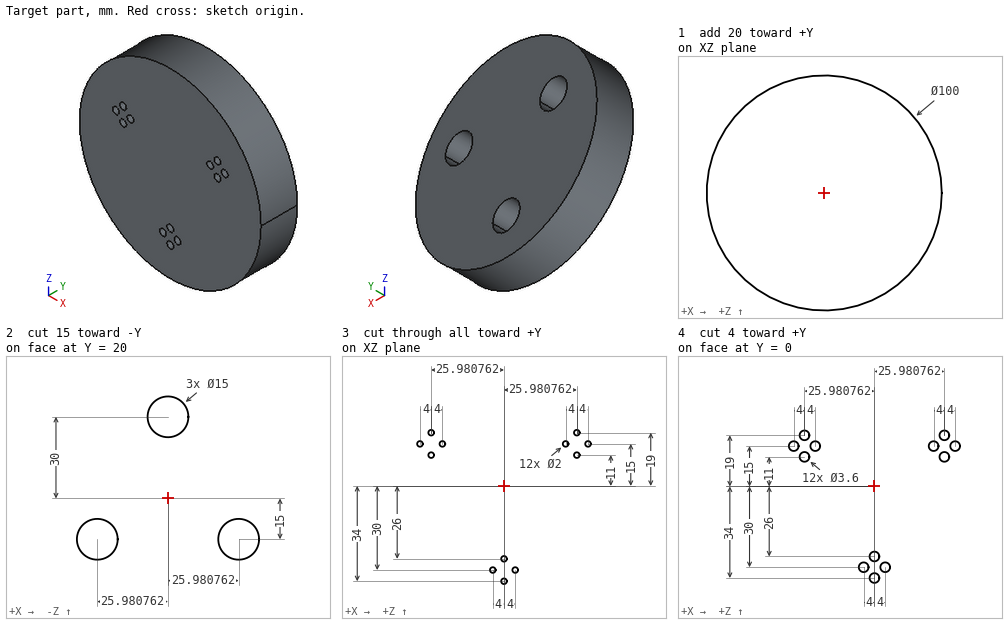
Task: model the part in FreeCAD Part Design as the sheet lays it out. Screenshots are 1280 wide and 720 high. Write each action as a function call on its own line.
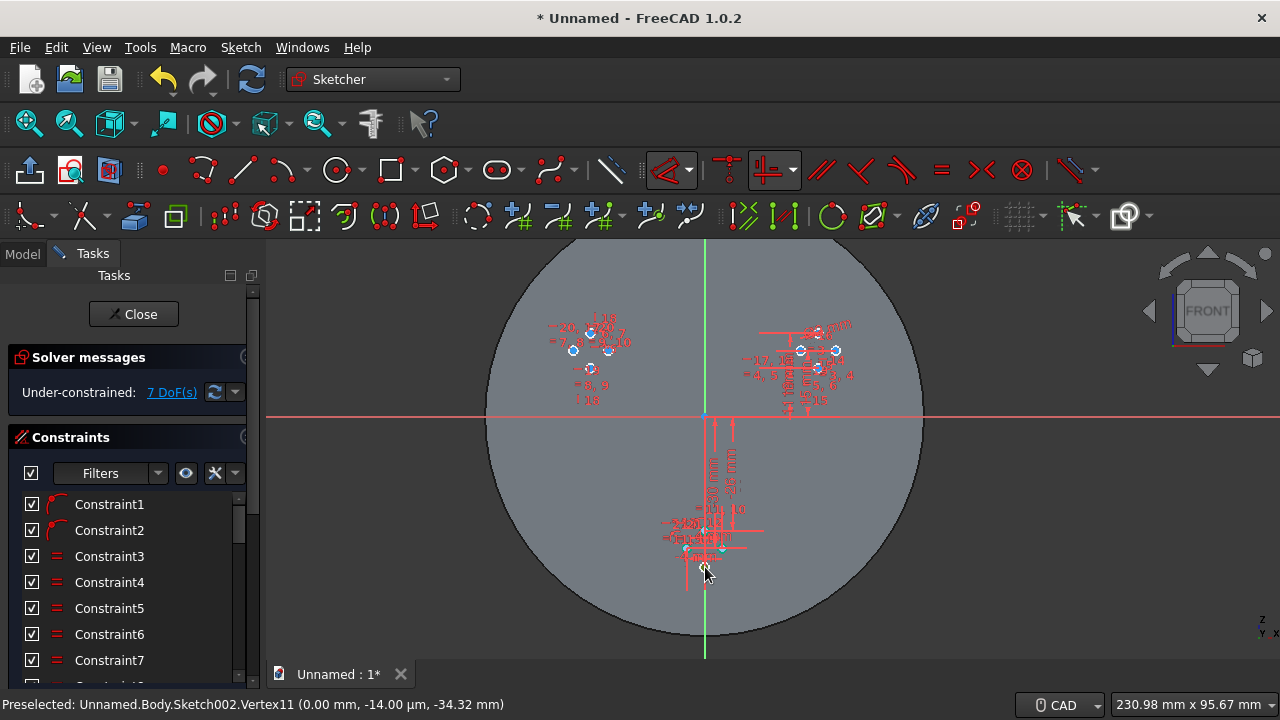
key(i)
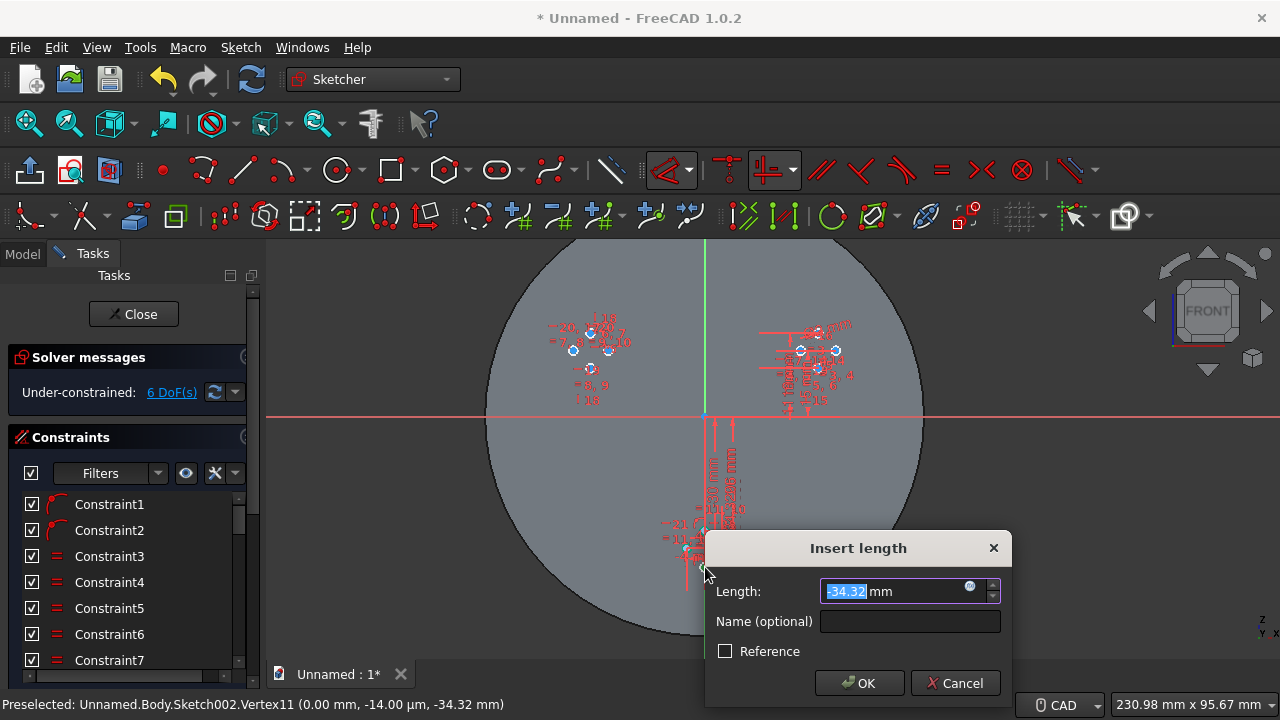
text(-34)
key(Return)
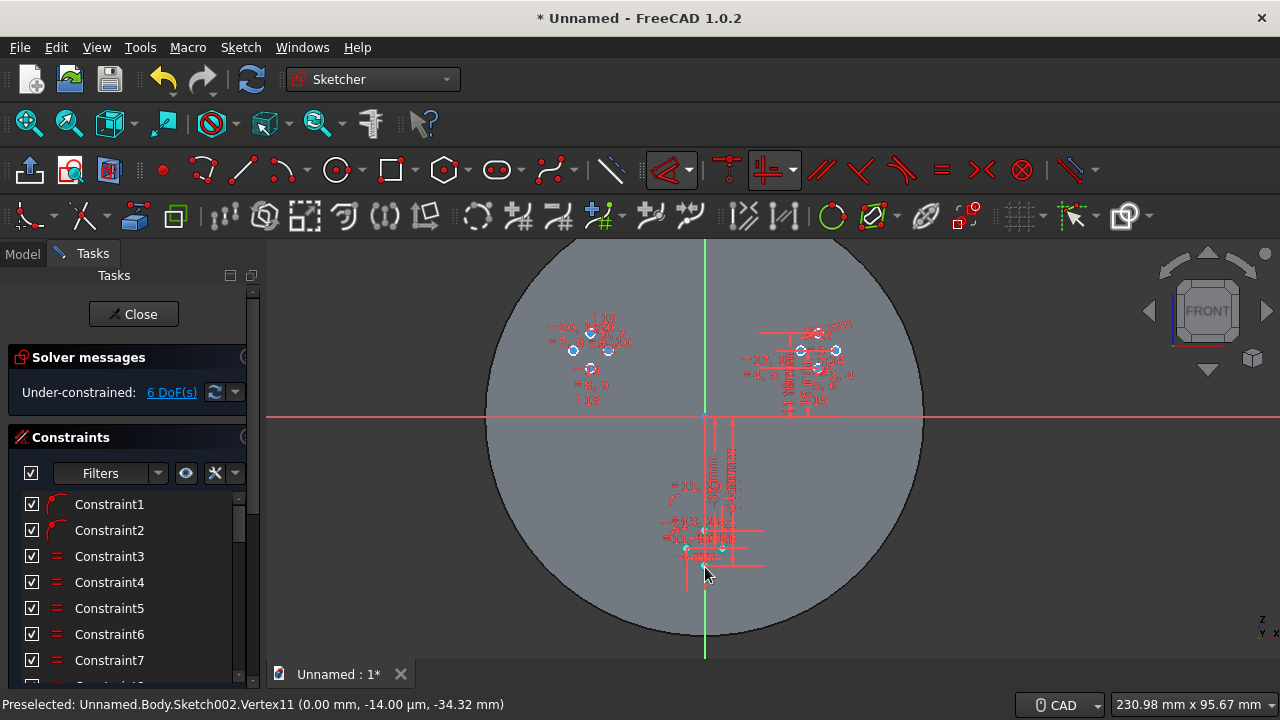
scroll(818, 333, up, 5)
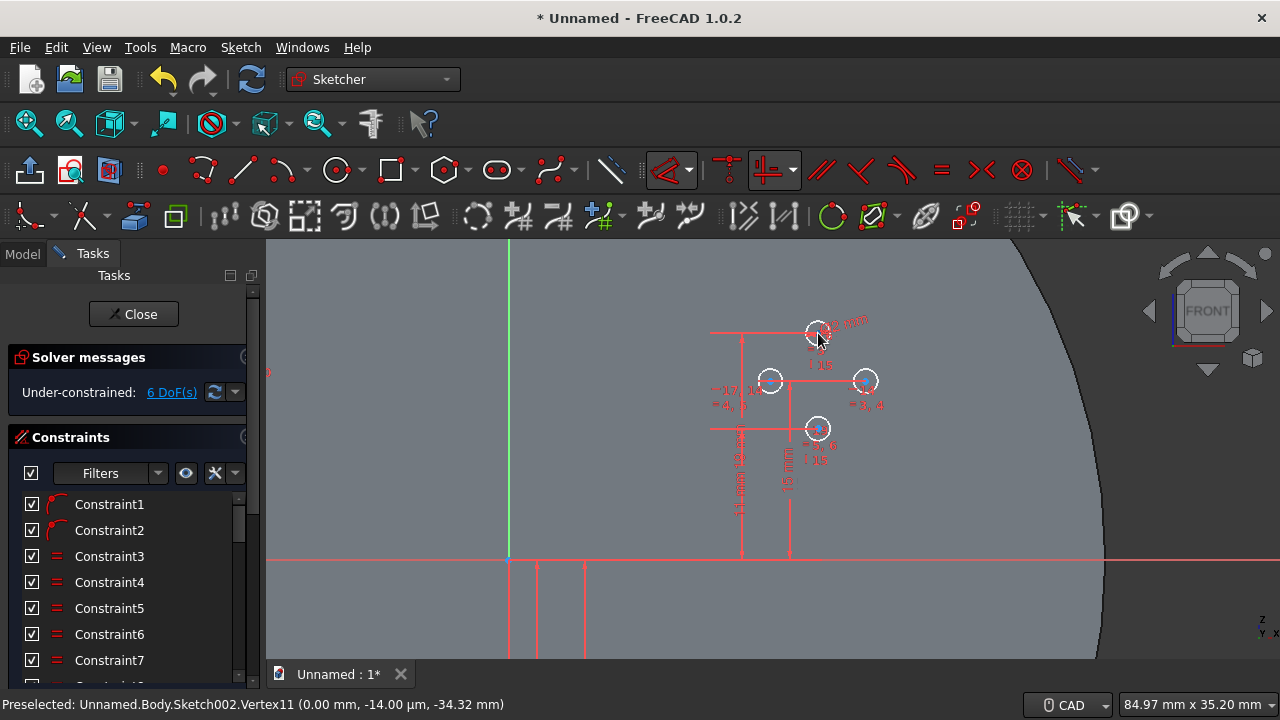
click(818, 333)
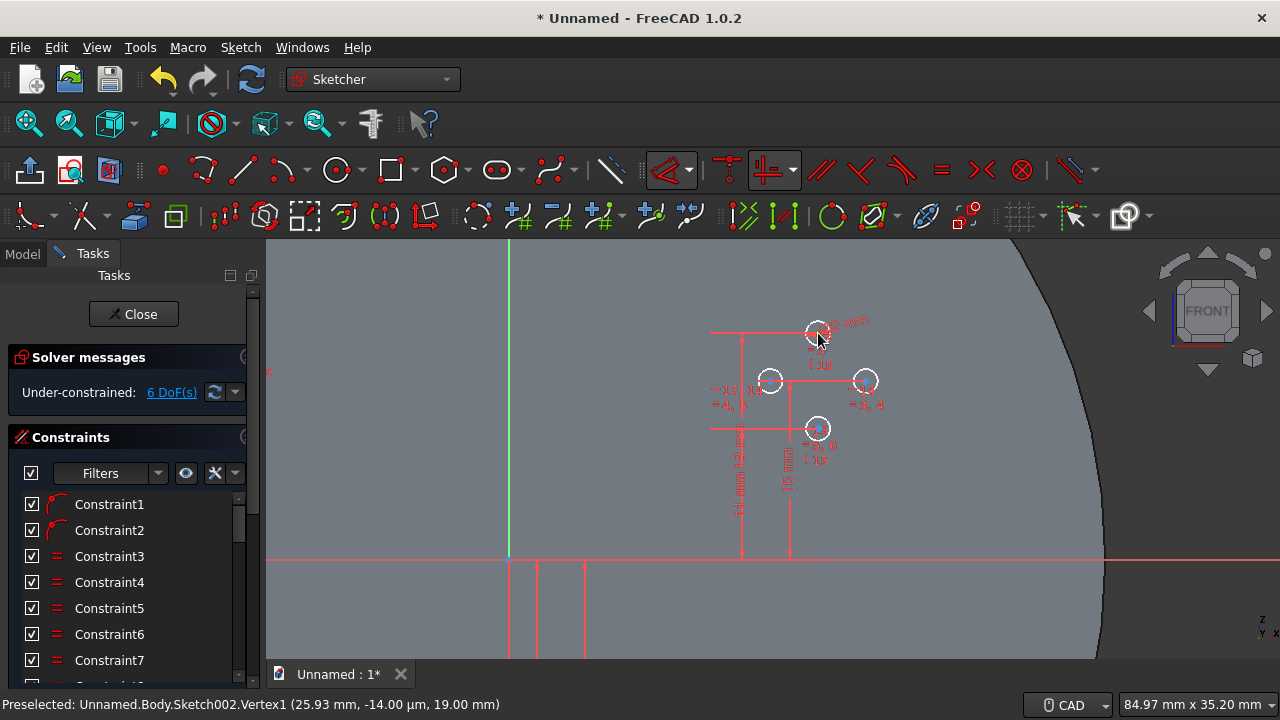
click(866, 381)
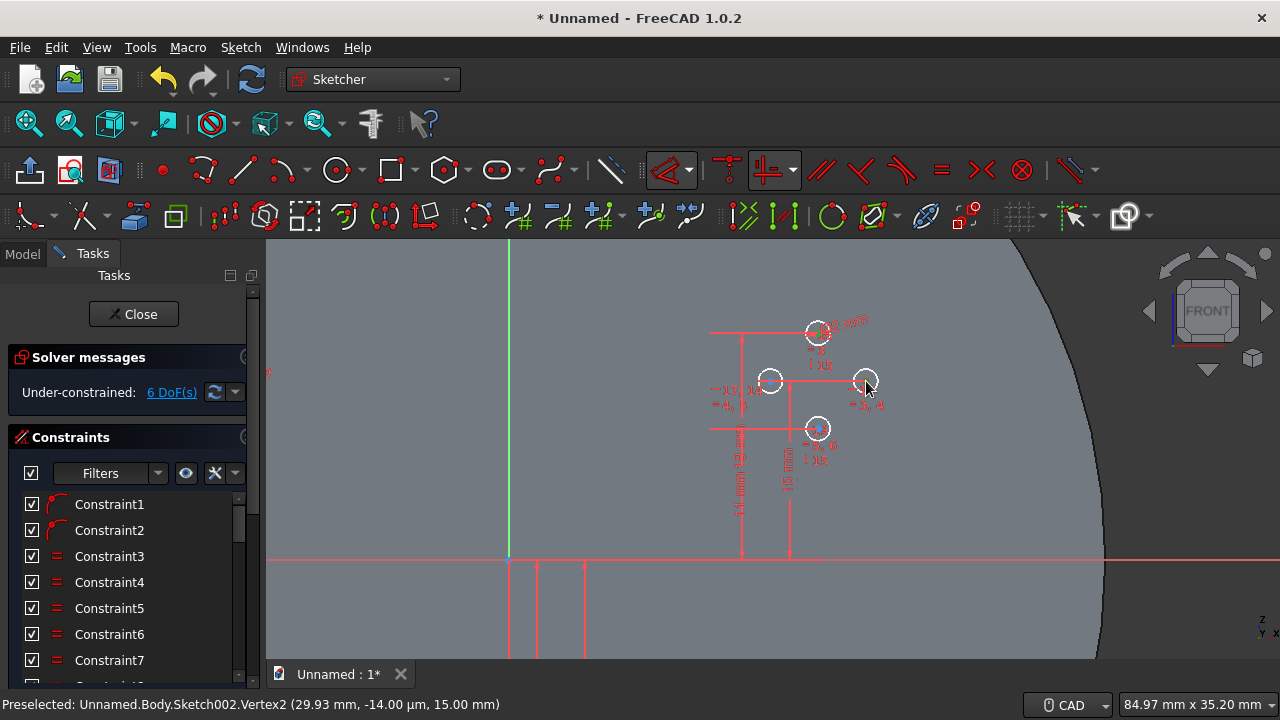
click(692, 170)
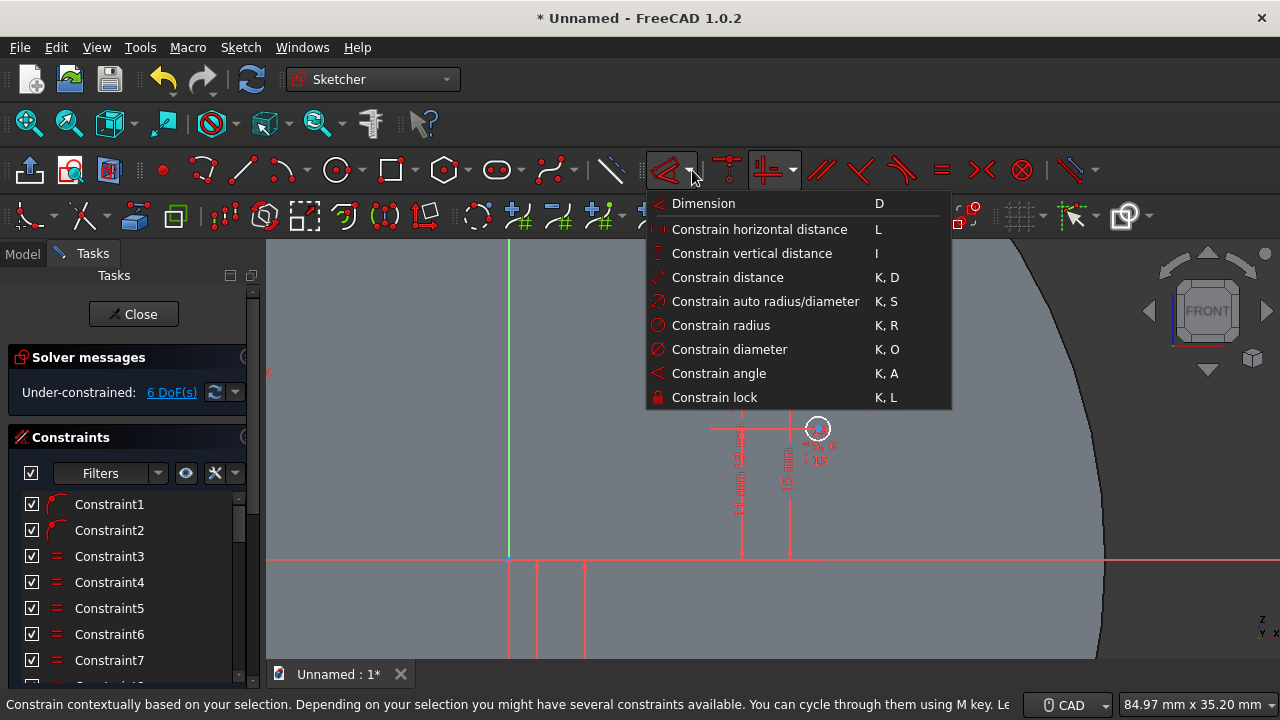
click(799, 229)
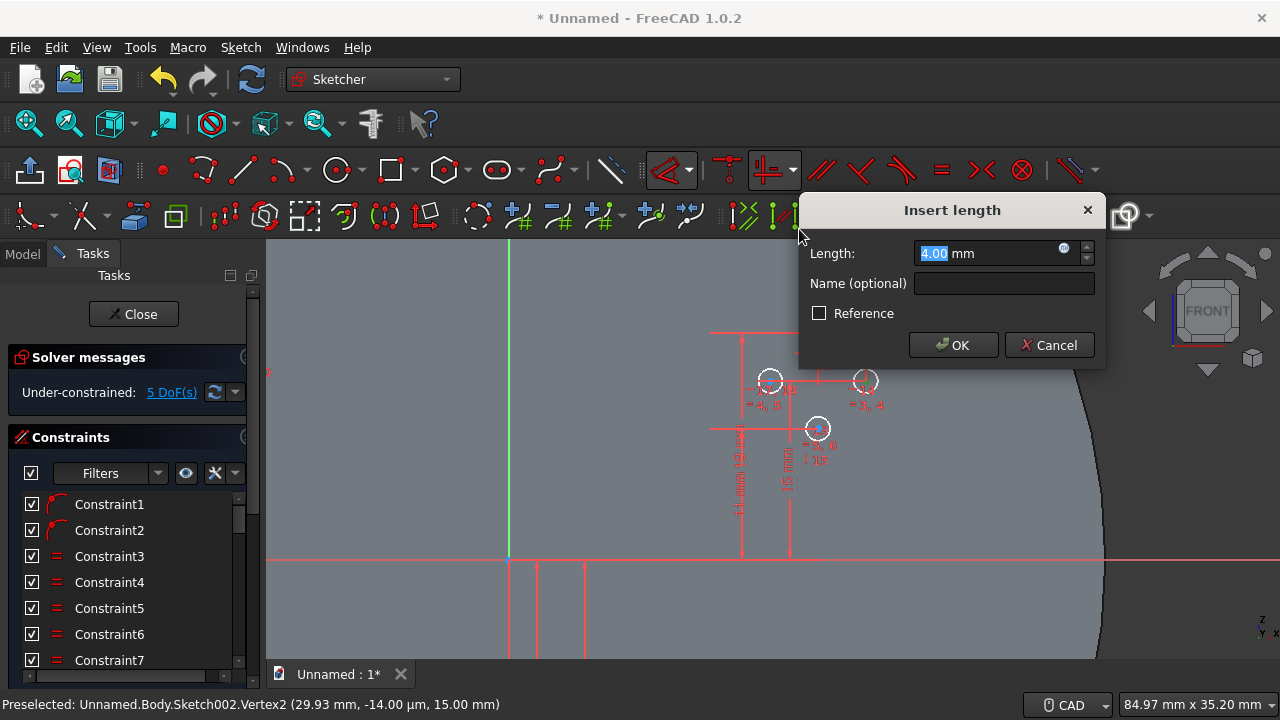
text(4)
key(Return)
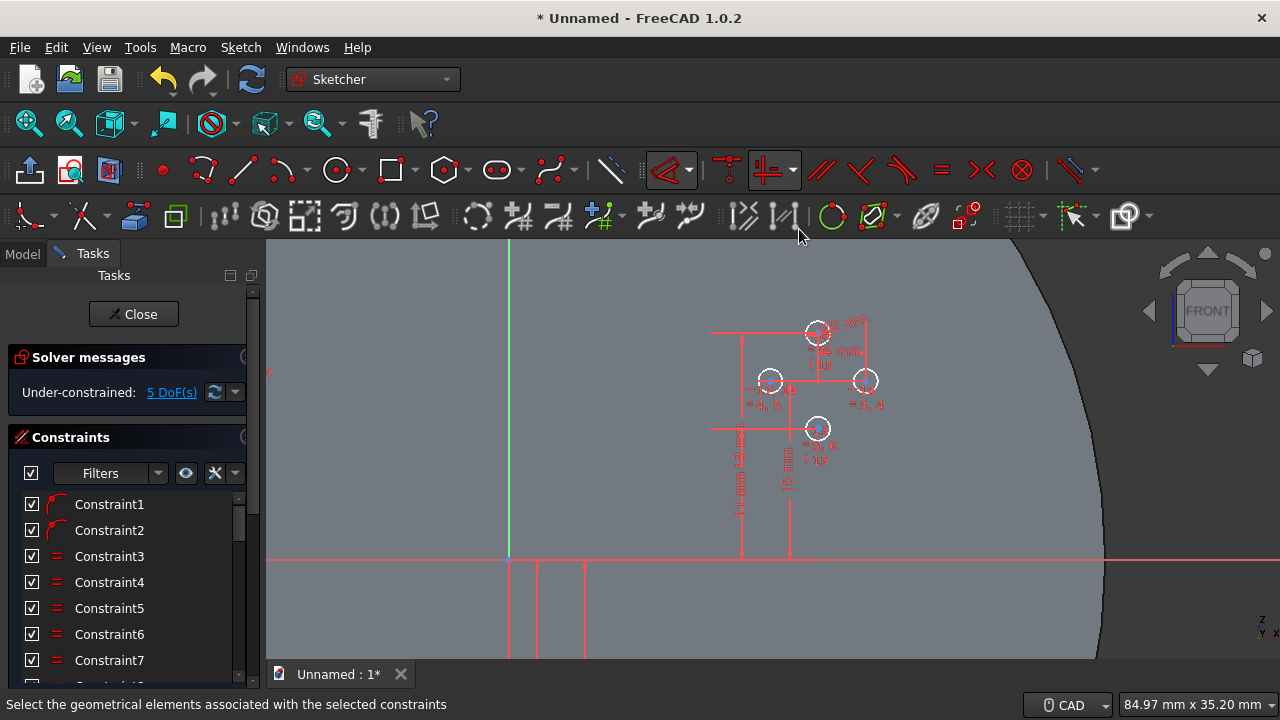
click(818, 333)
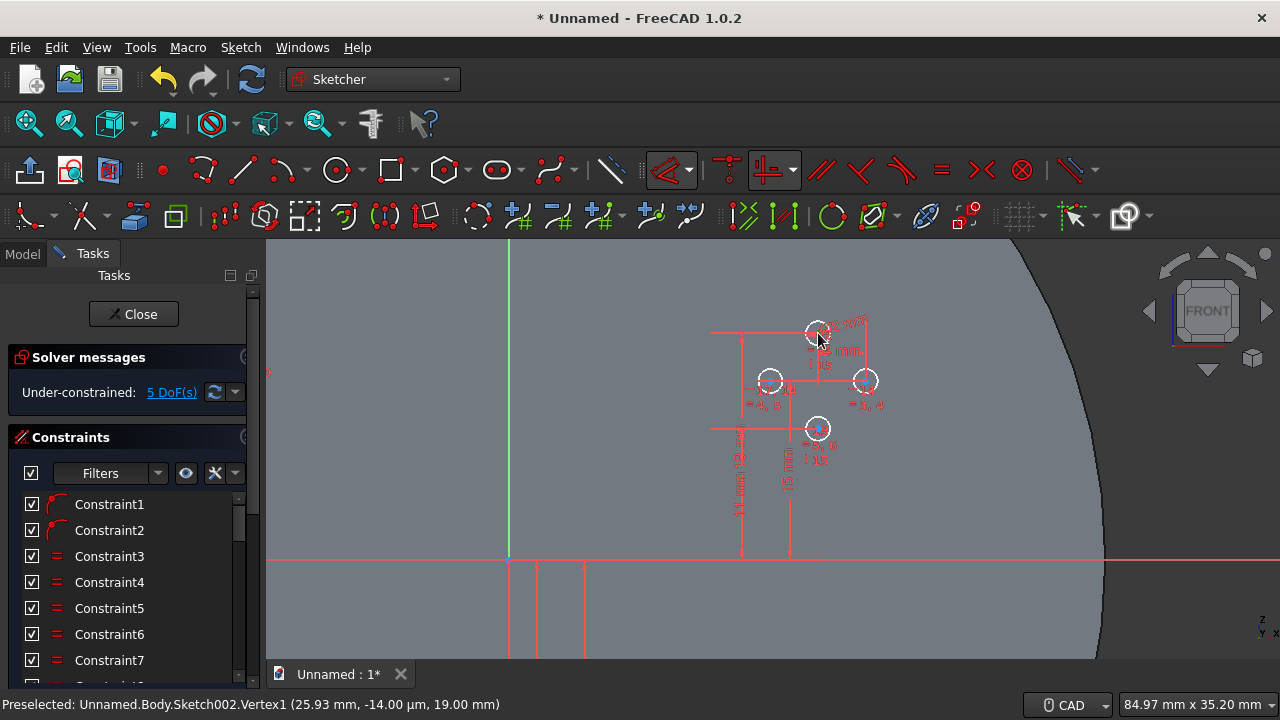
click(770, 381)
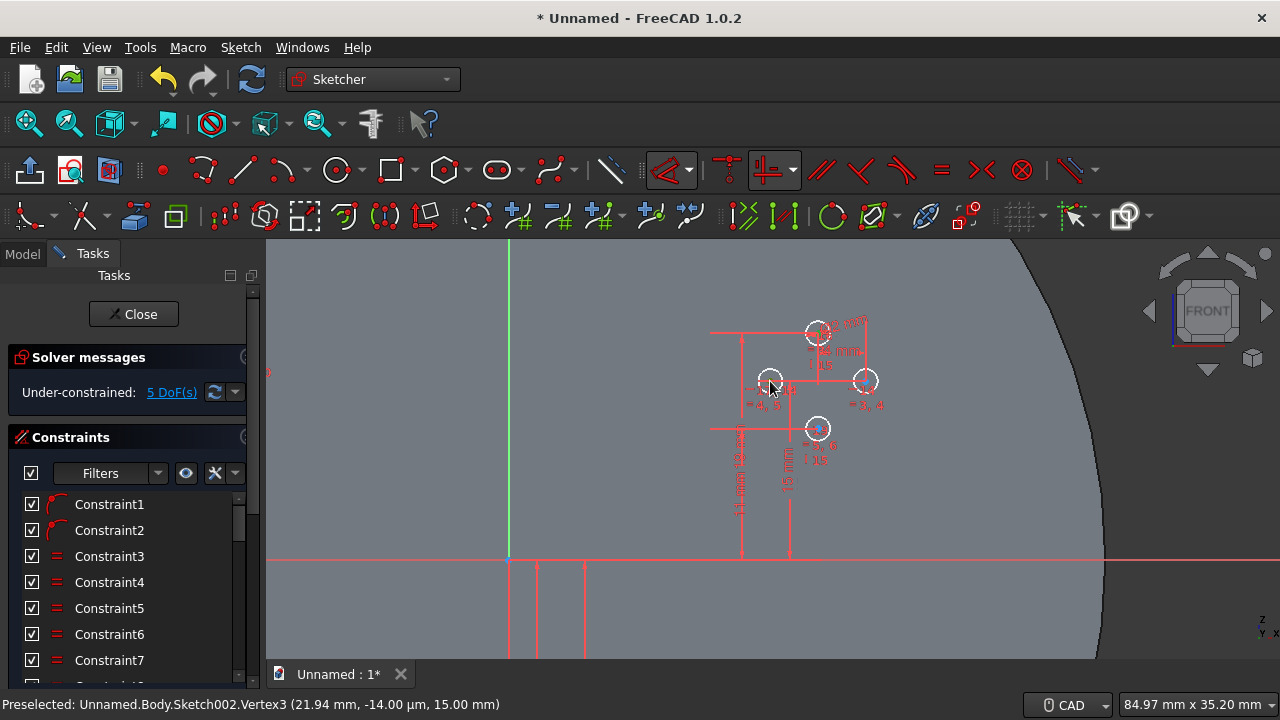
click(692, 170)